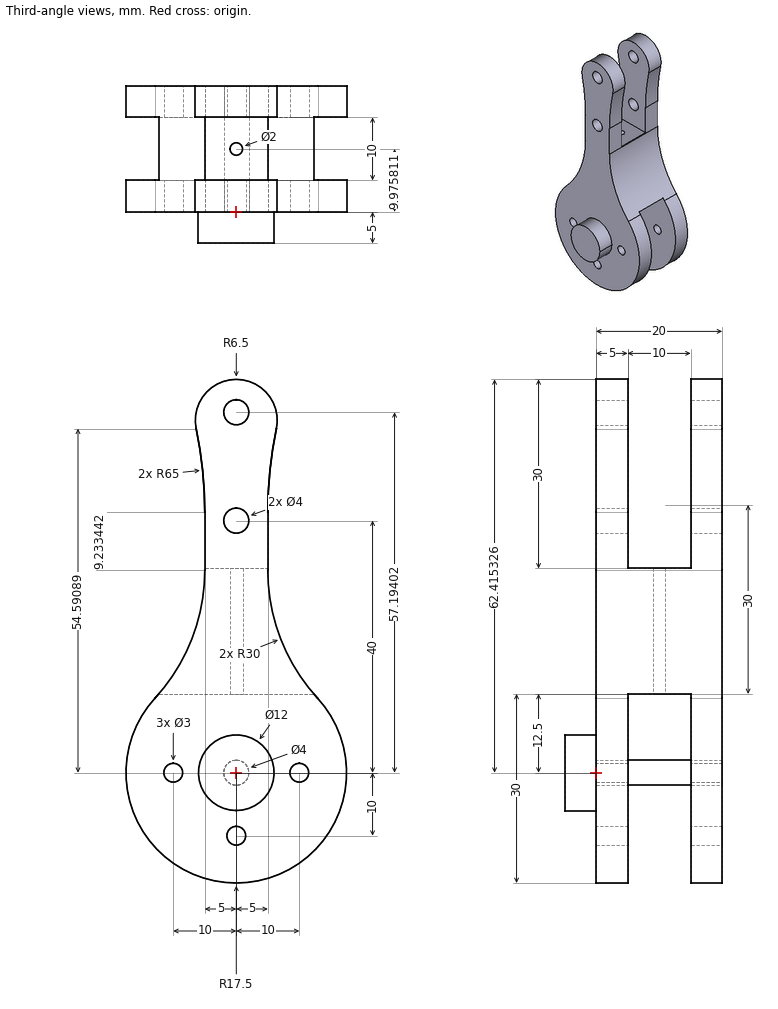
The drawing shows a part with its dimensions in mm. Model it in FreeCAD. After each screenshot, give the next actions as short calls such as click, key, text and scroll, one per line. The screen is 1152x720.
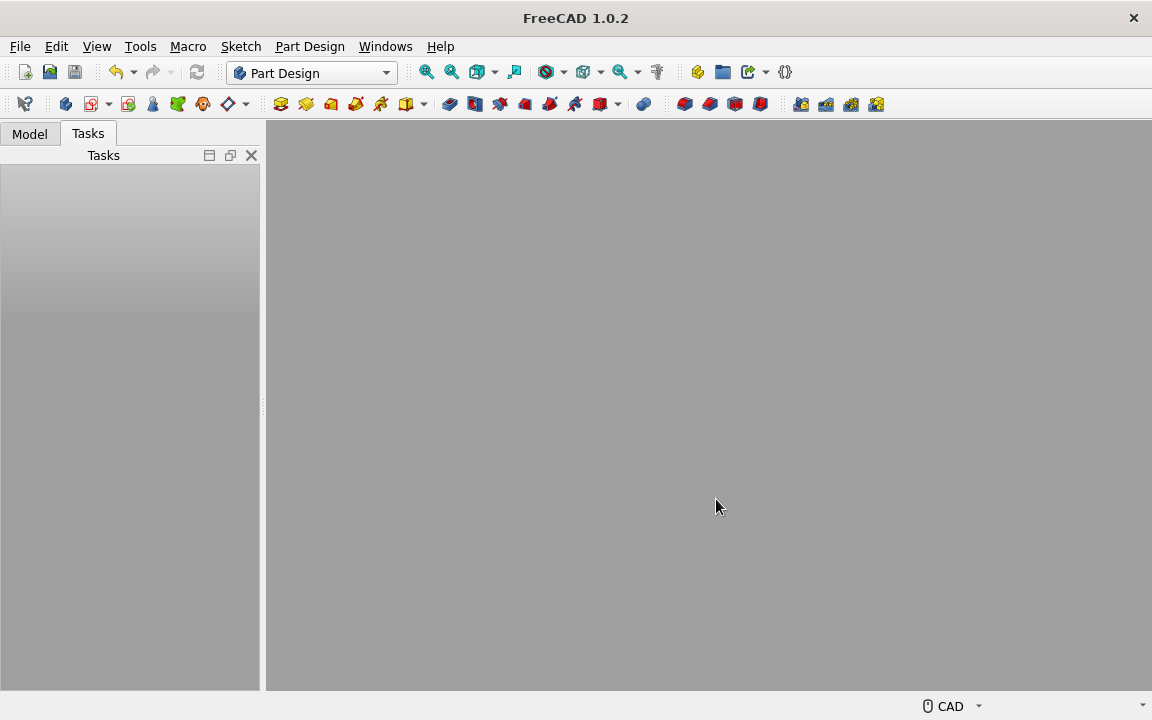
click(25, 72)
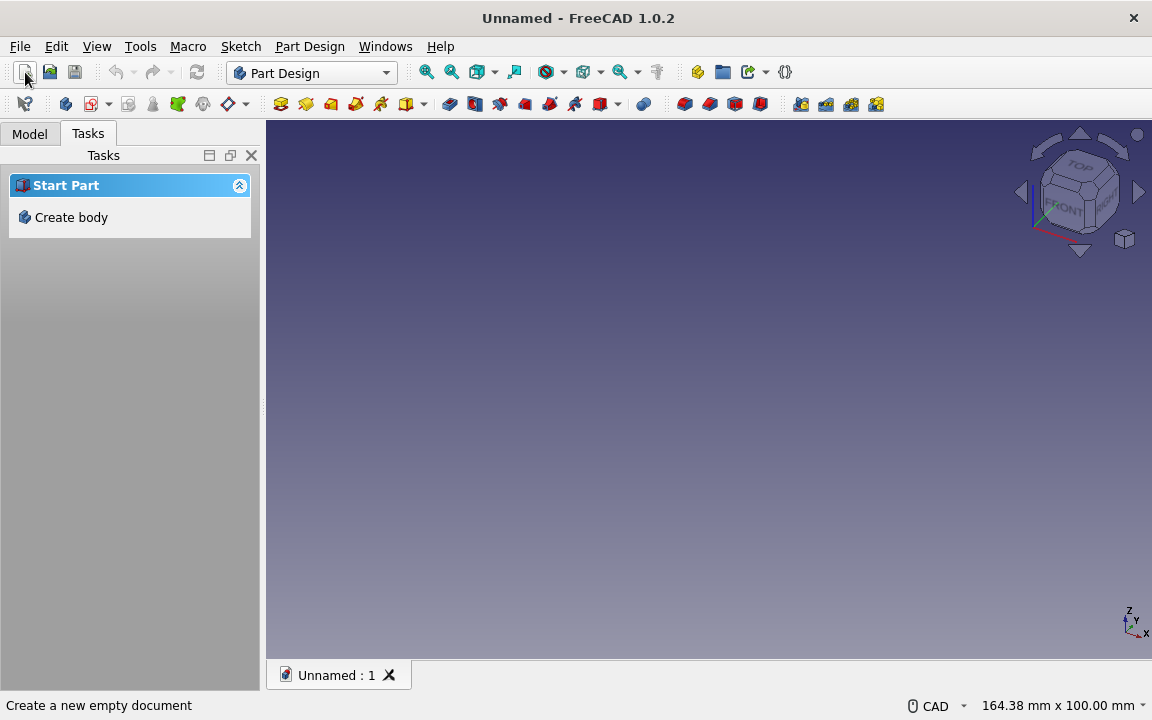
click(90, 104)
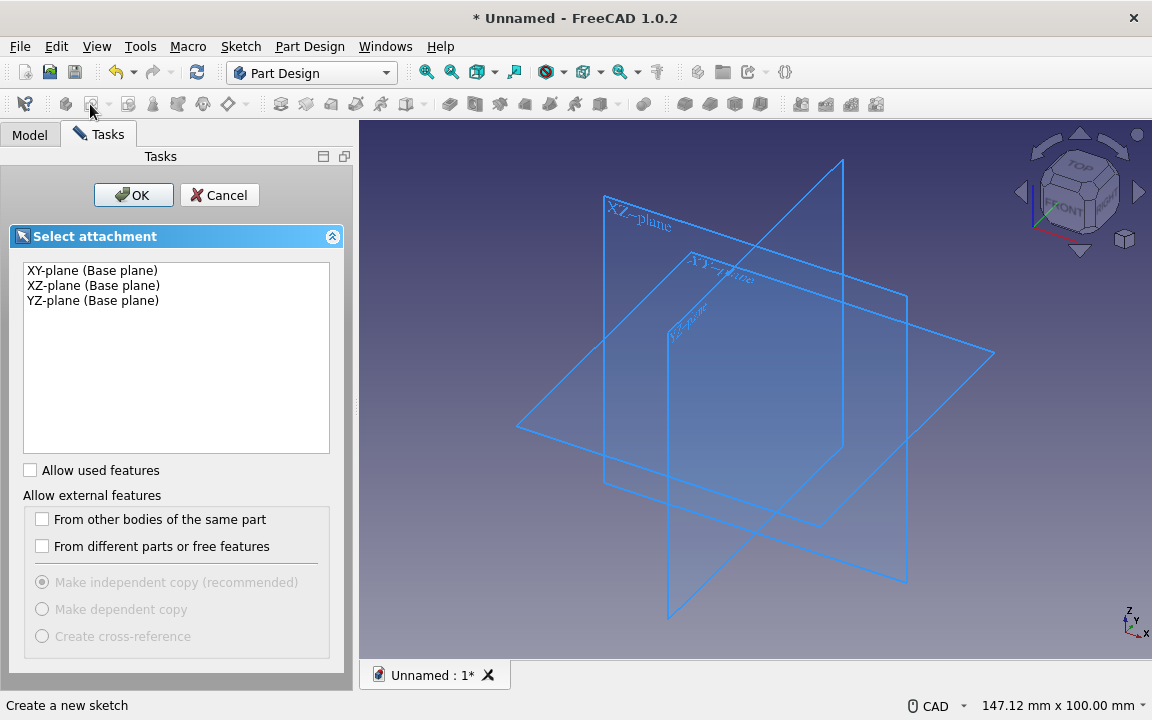
click(84, 286)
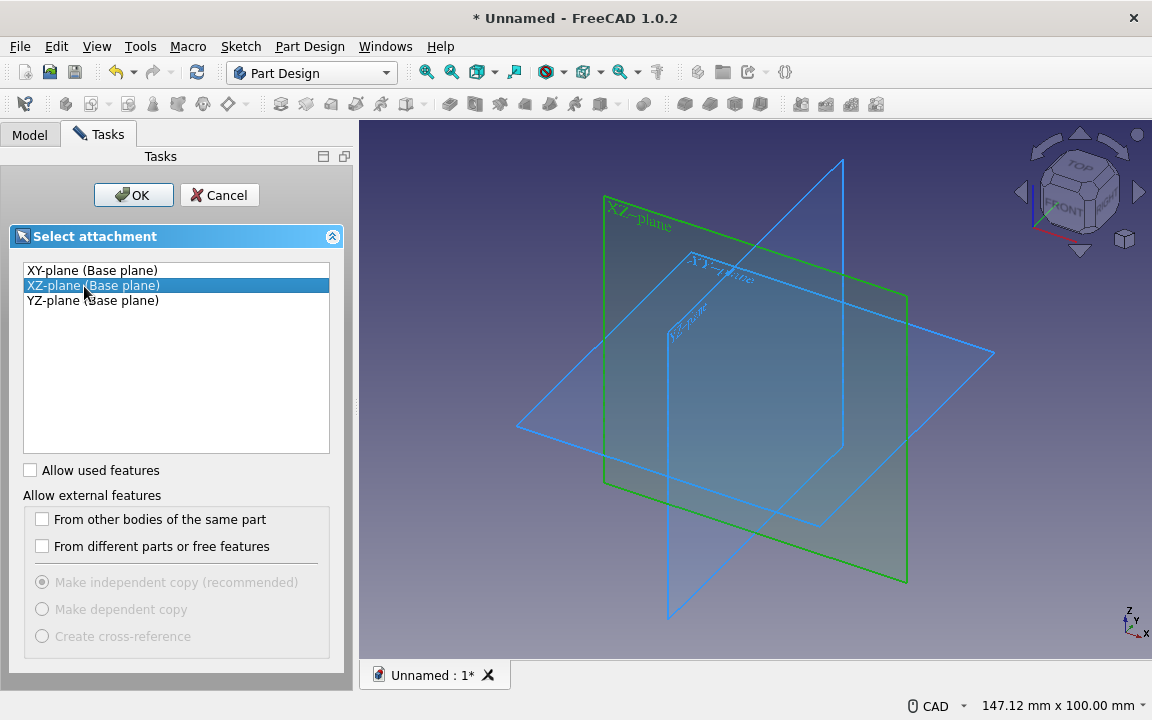
click(134, 195)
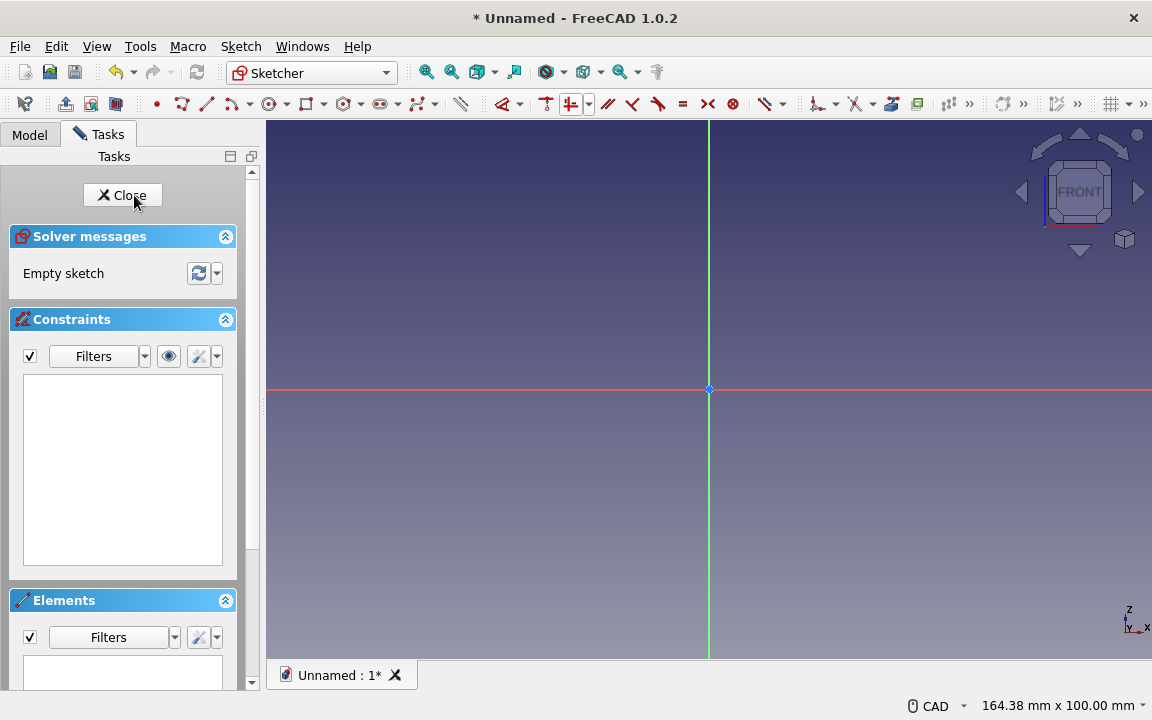
scroll(501, 631, down, 2)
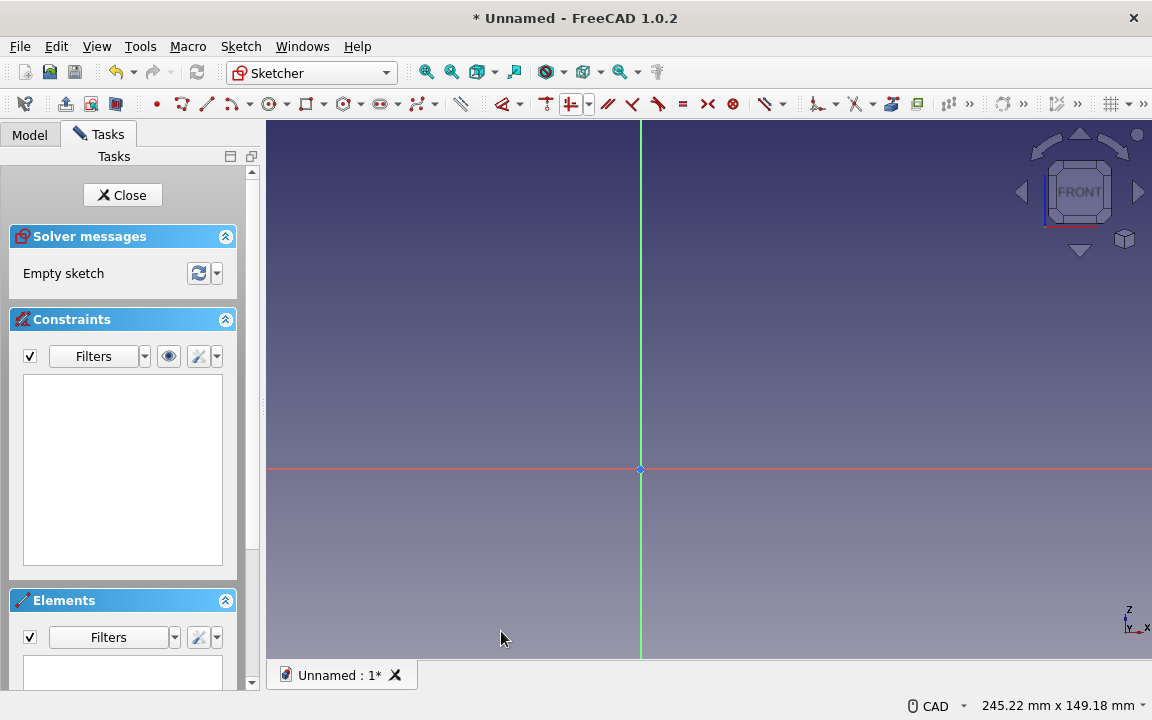
click(207, 104)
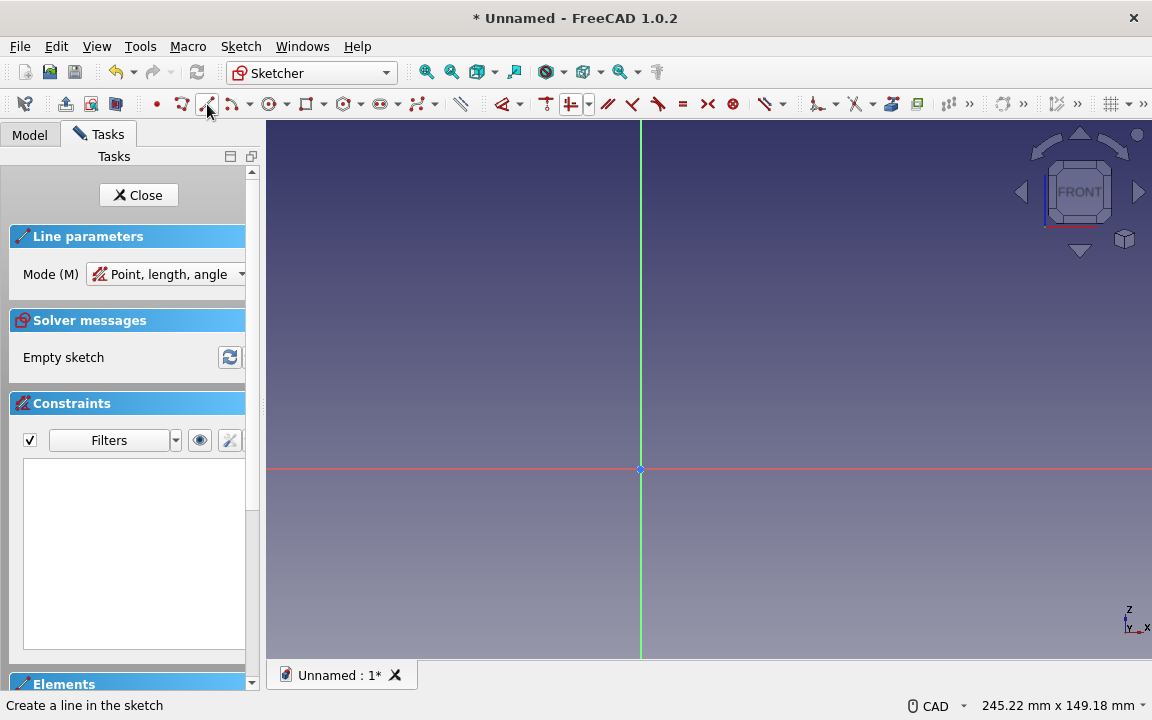
click(622, 353)
click(622, 320)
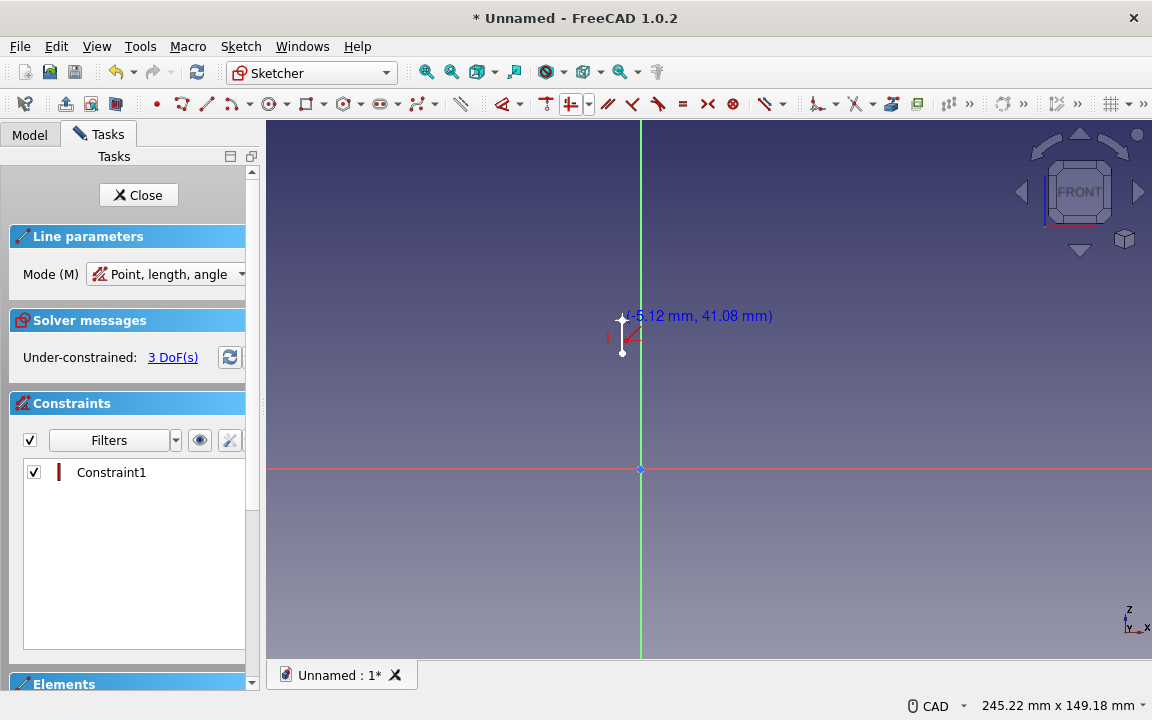
click(659, 320)
click(659, 353)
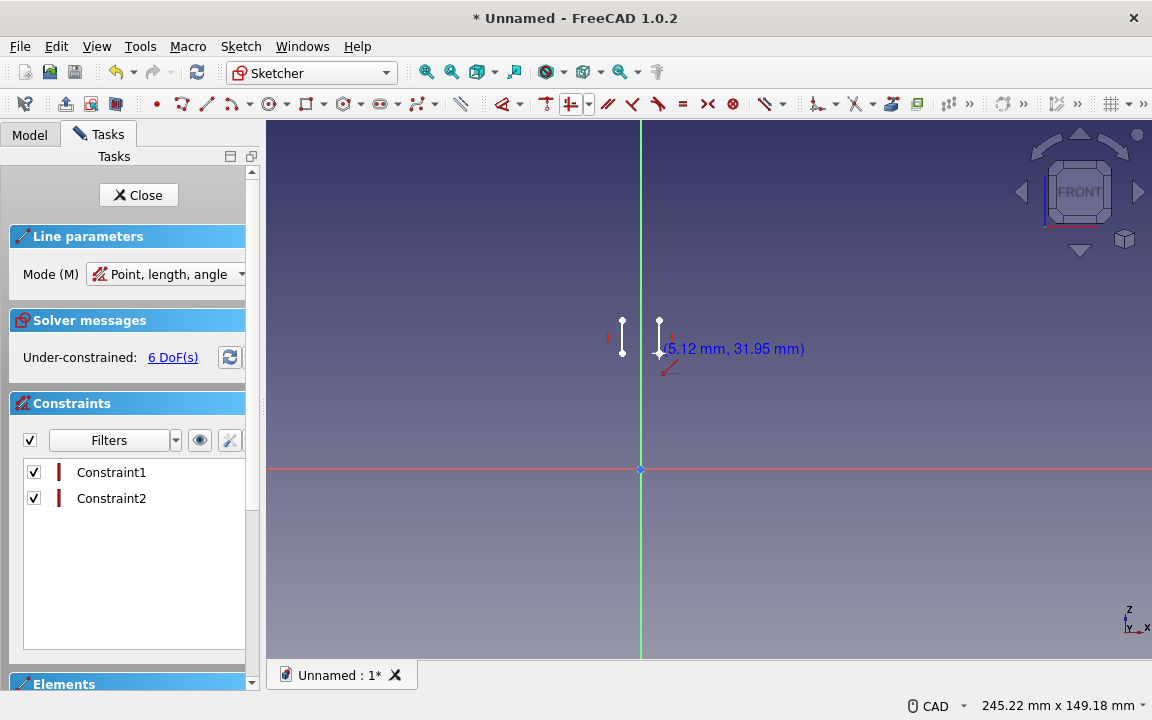
key(g)
key(3)
key(a)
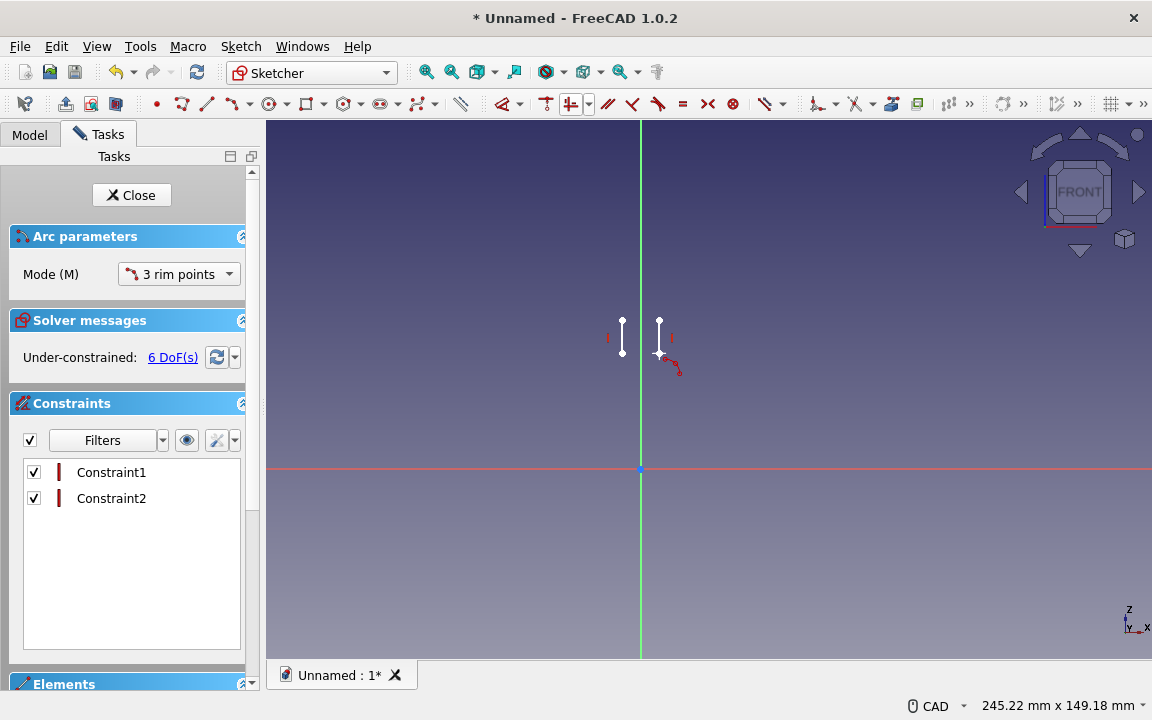
click(622, 321)
click(618, 272)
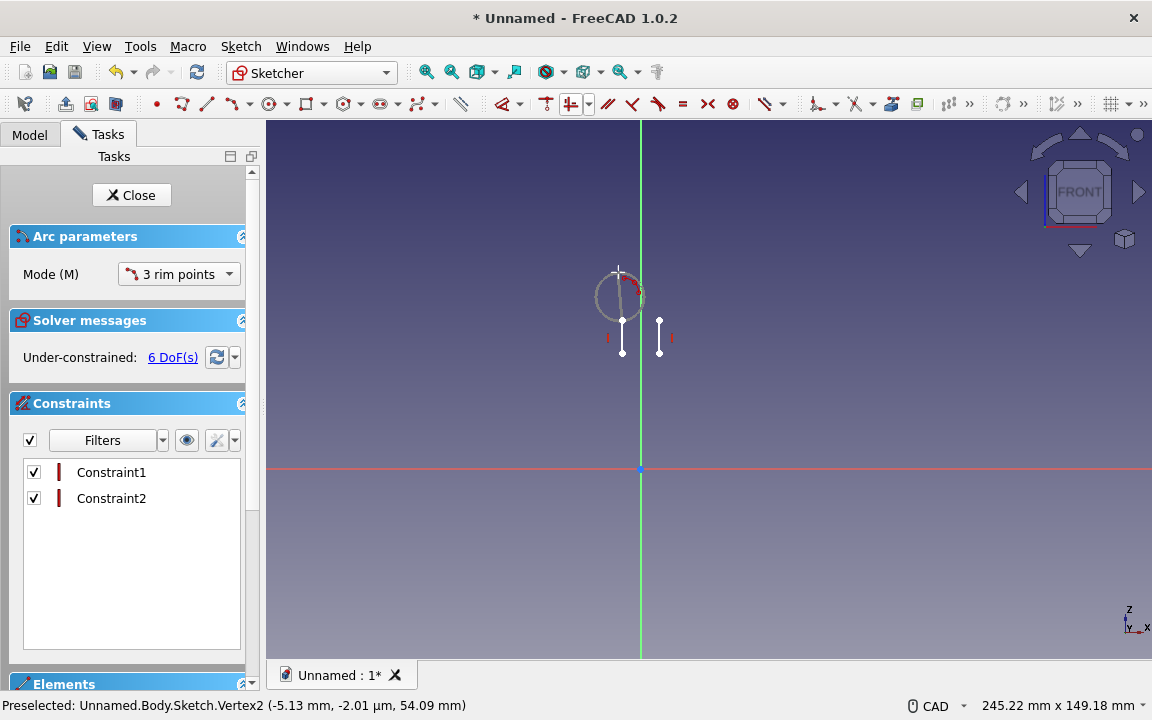
scroll(621, 296, up, 13)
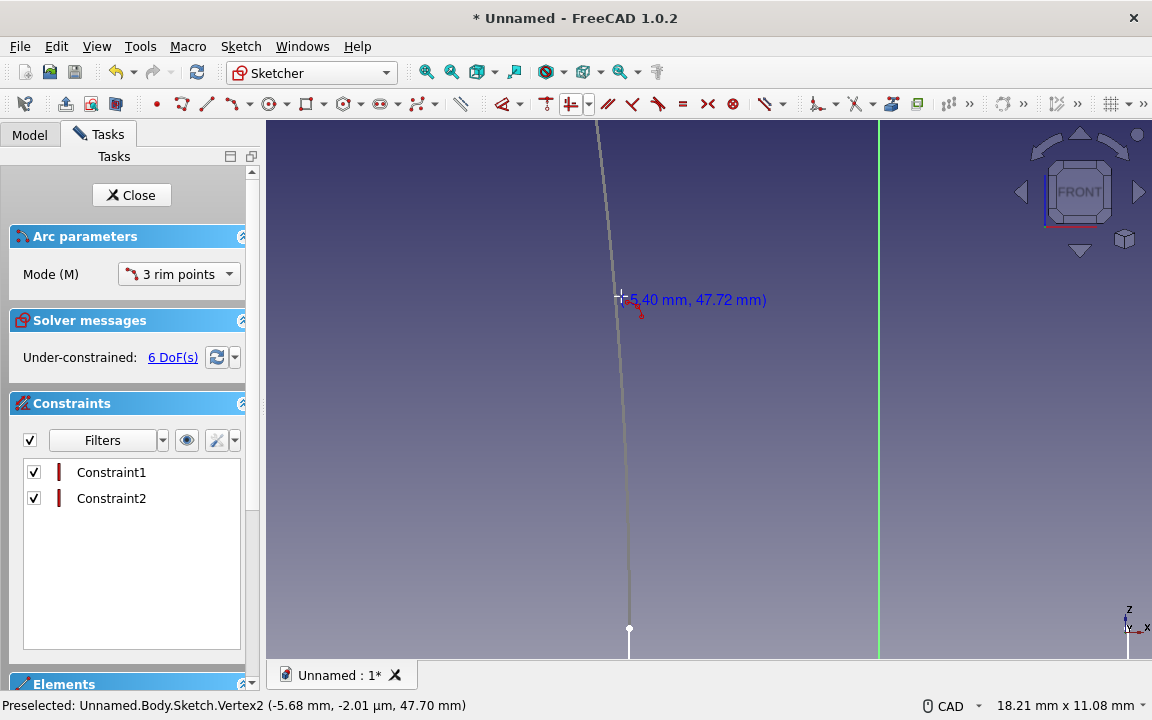
click(619, 292)